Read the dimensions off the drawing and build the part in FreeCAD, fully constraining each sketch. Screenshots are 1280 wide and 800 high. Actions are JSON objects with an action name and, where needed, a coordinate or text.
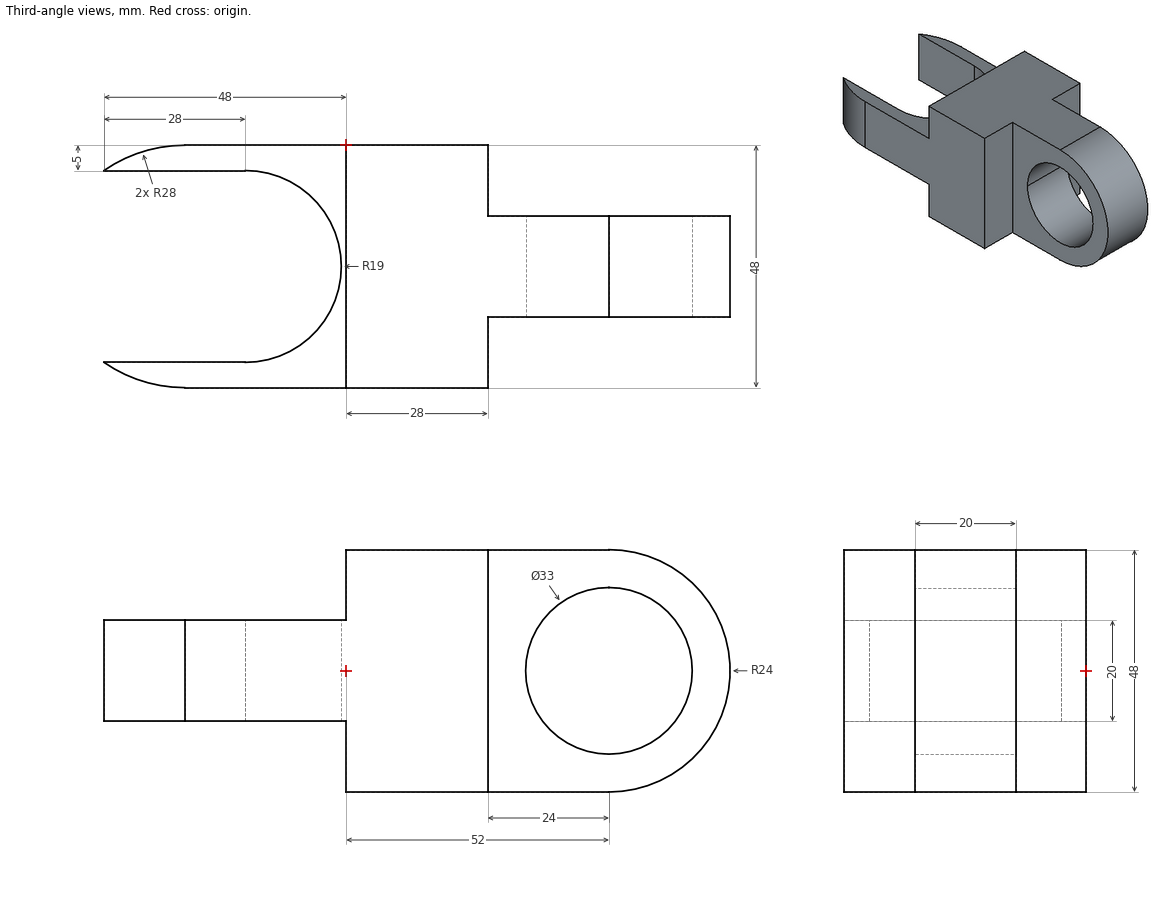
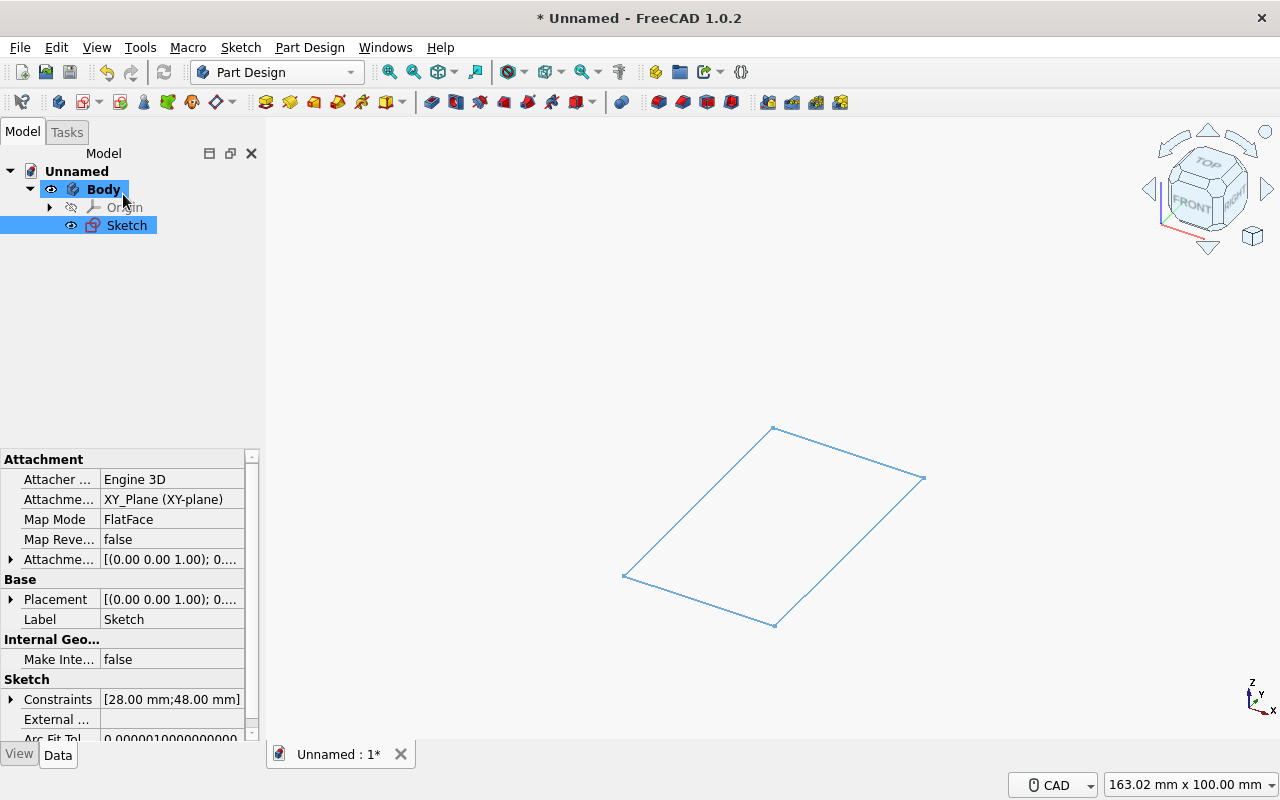
{"action": "left_click", "coordinate": [266, 102]}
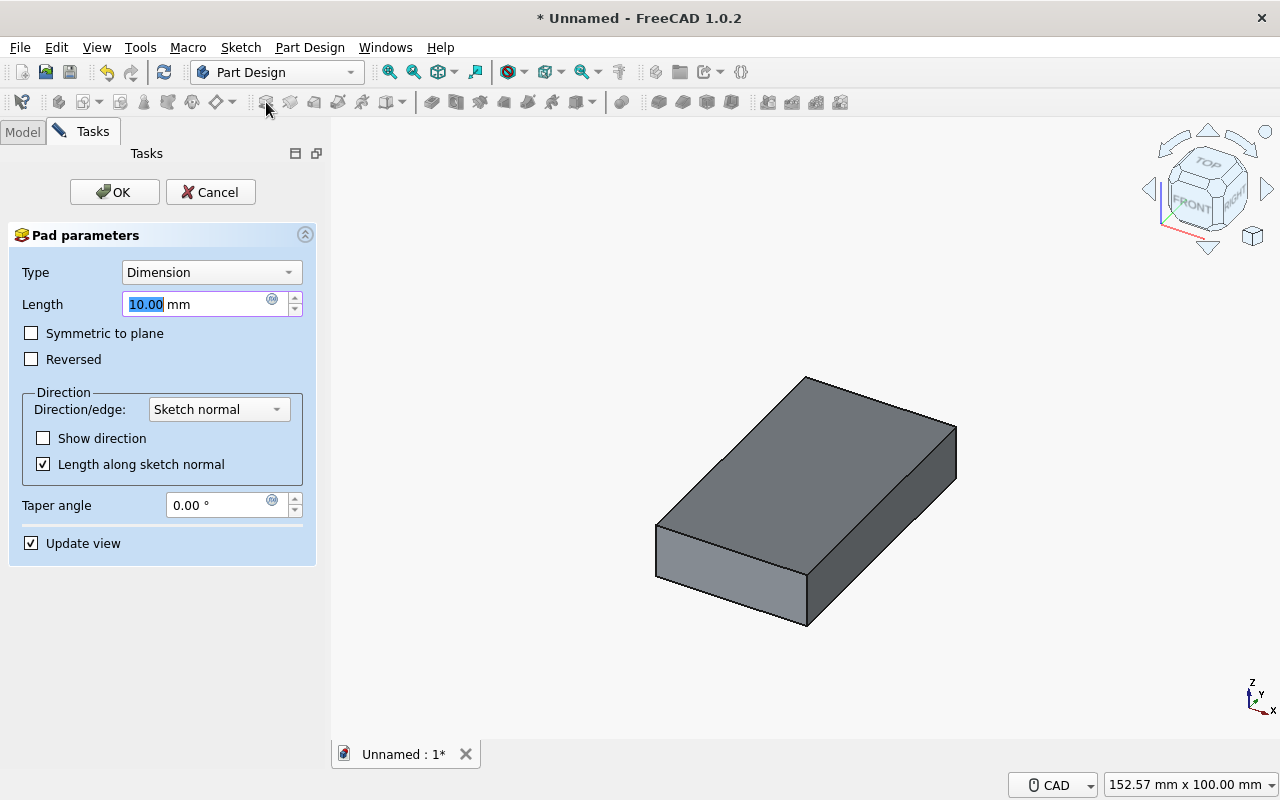
{"action": "type", "text": "48"}
{"action": "key", "text": "Tab"}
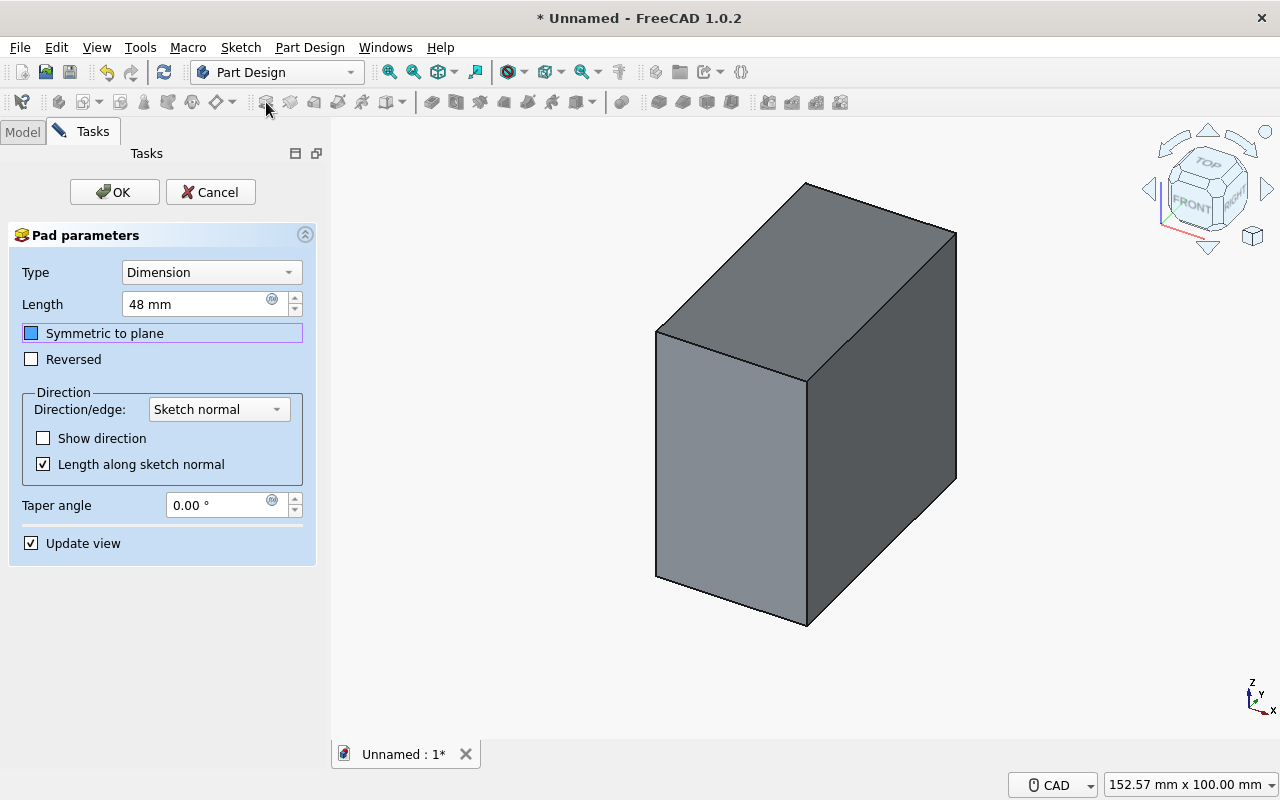
{"action": "left_click", "coordinate": [30, 333]}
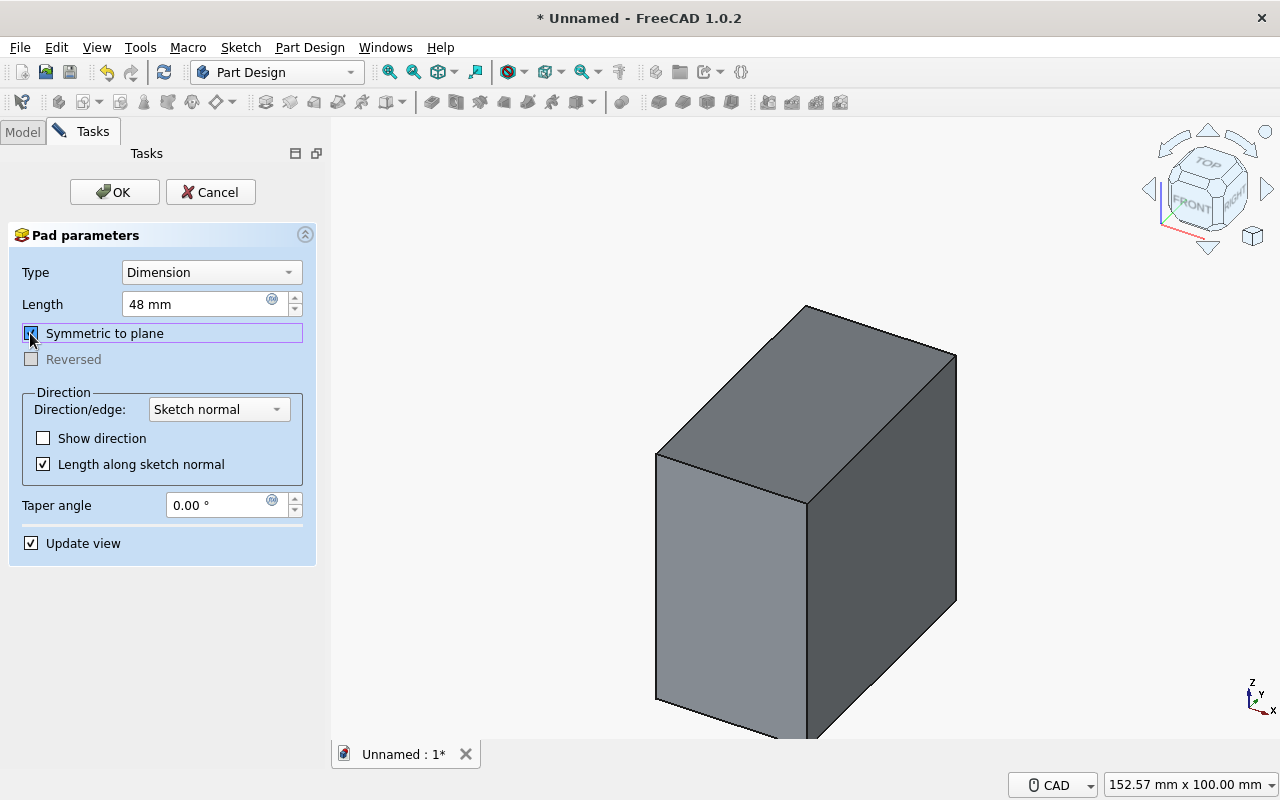
{"action": "left_click", "coordinate": [115, 192]}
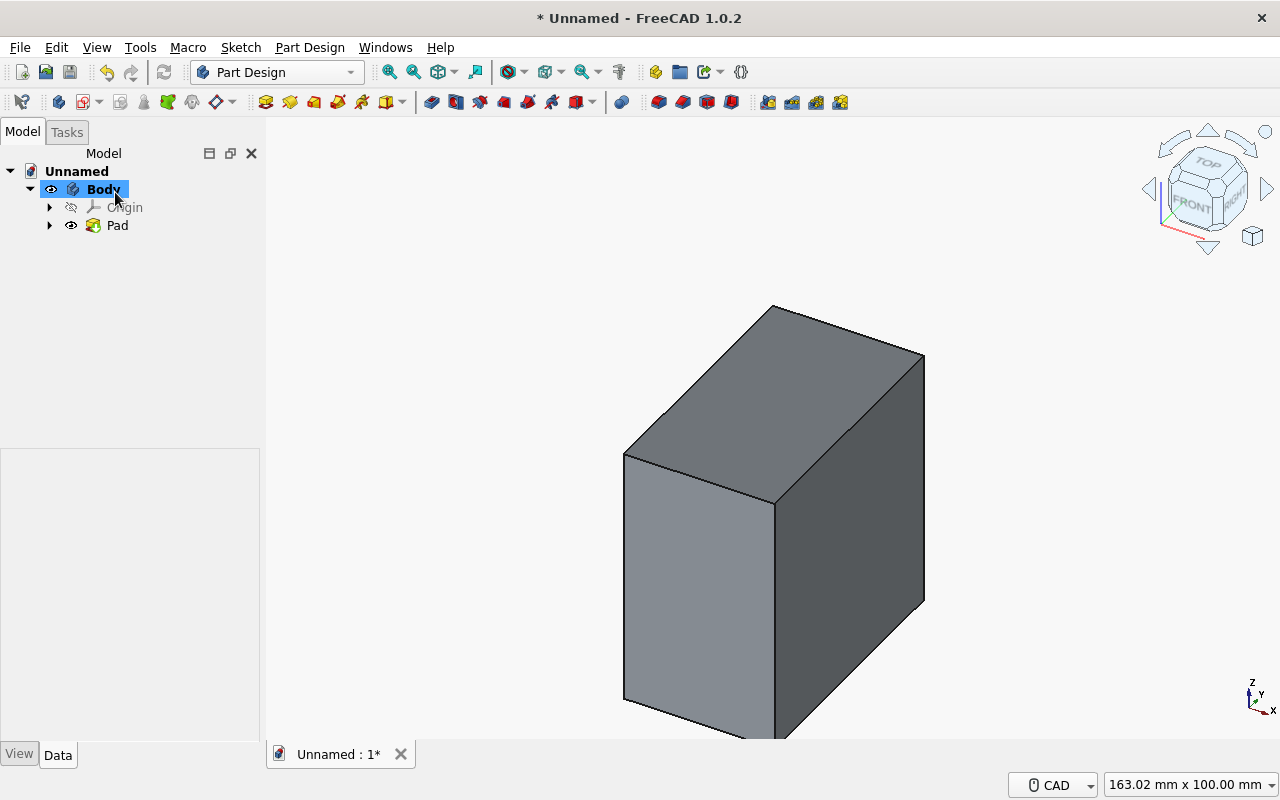
{"action": "left_click", "coordinate": [390, 72]}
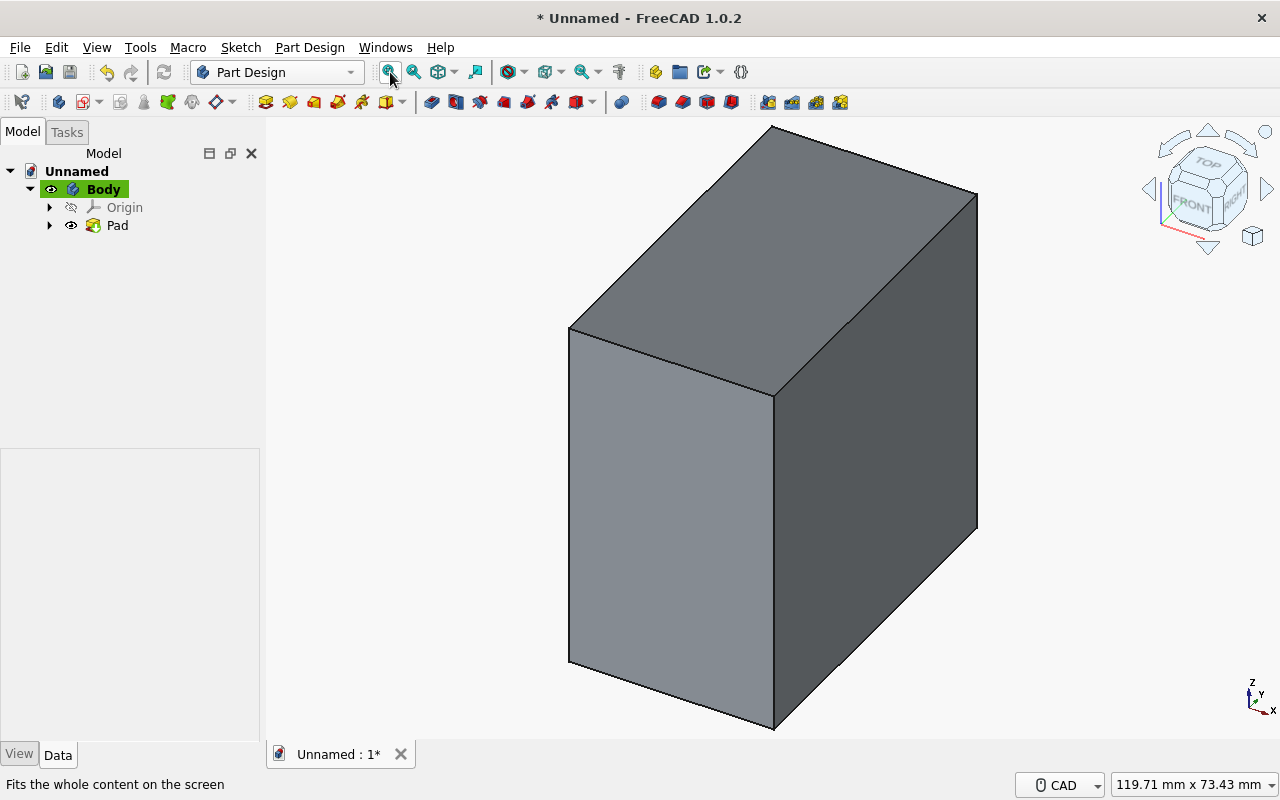
{"action": "left_click", "coordinate": [50, 207]}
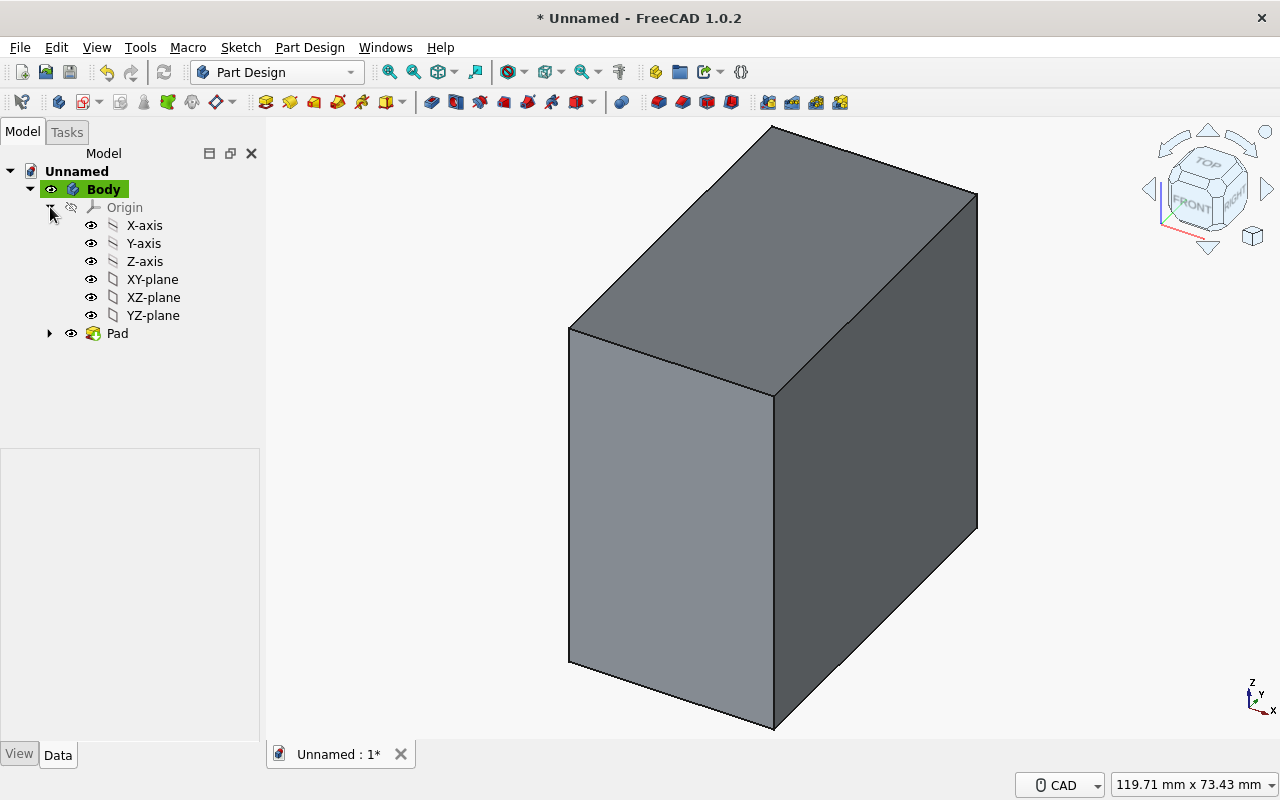
{"action": "left_click", "coordinate": [136, 297]}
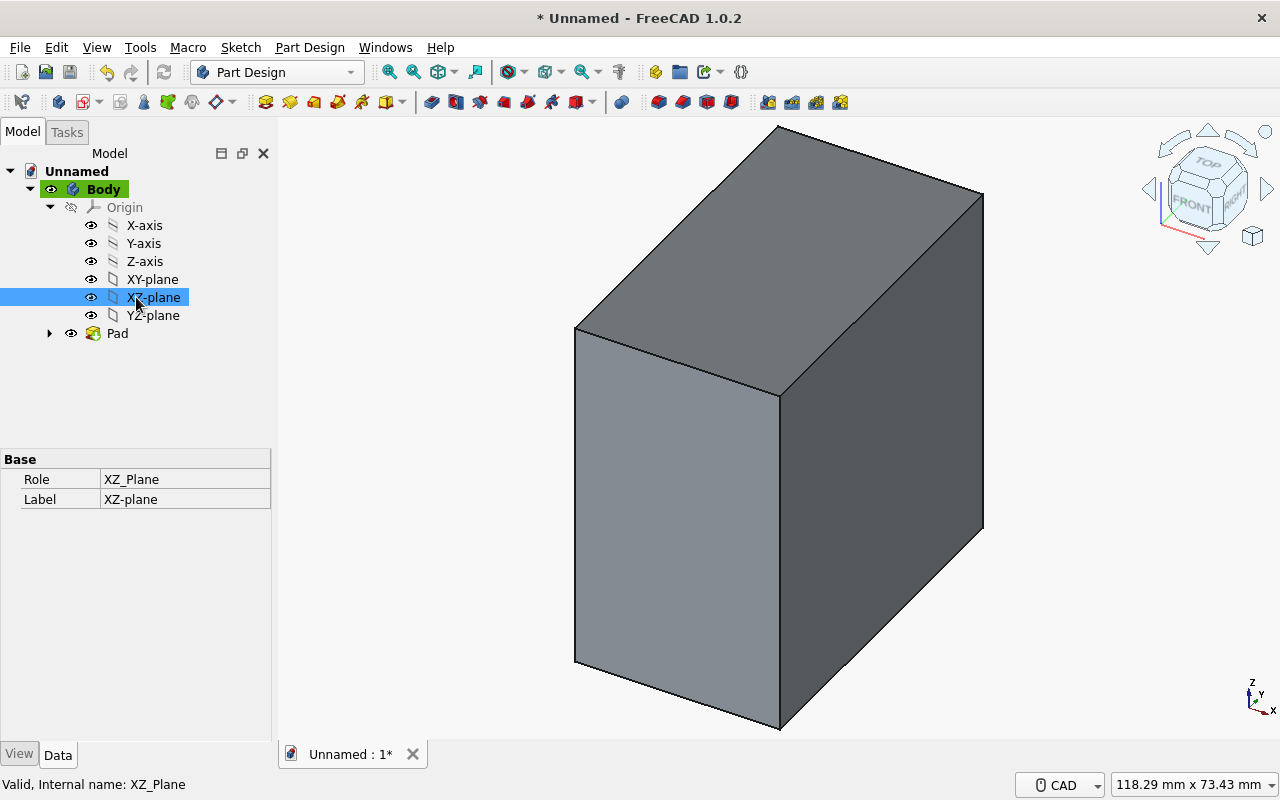
{"action": "left_click", "coordinate": [216, 102]}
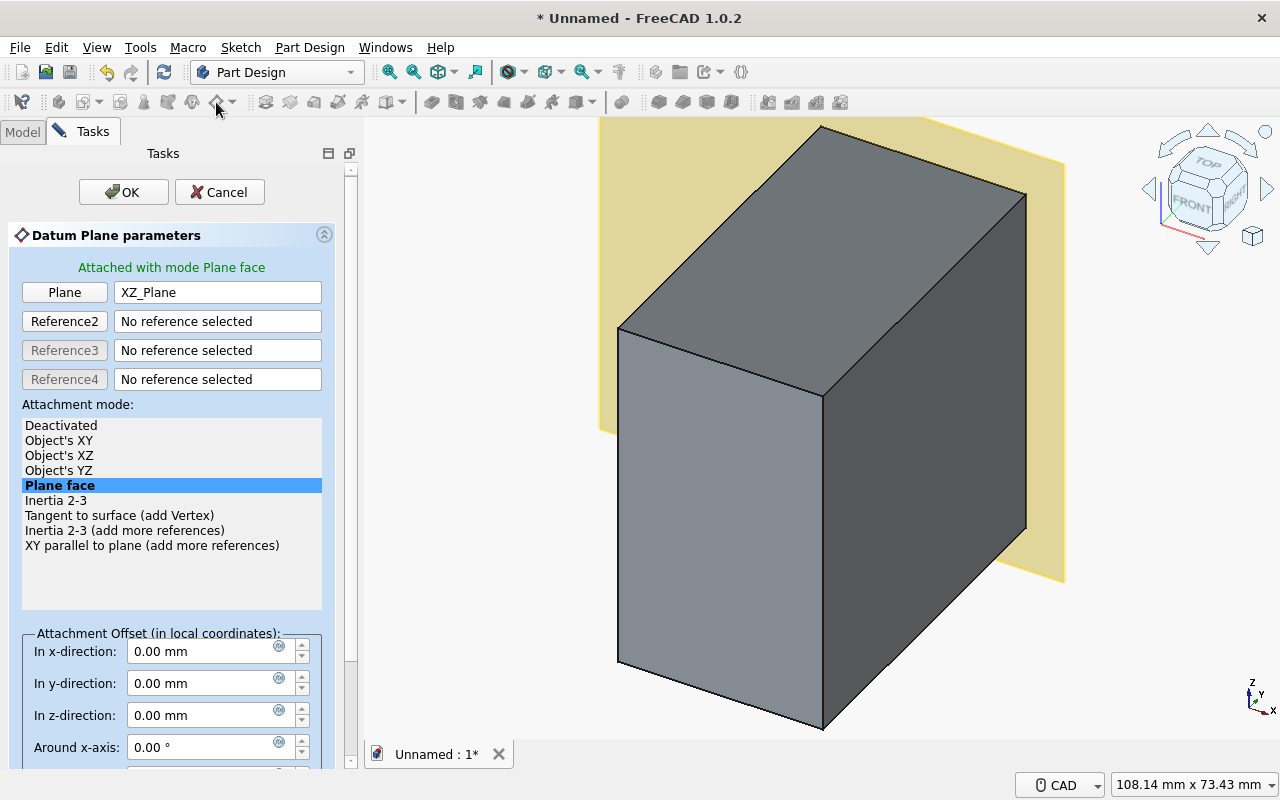
{"action": "triple_click", "coordinate": [210, 715]}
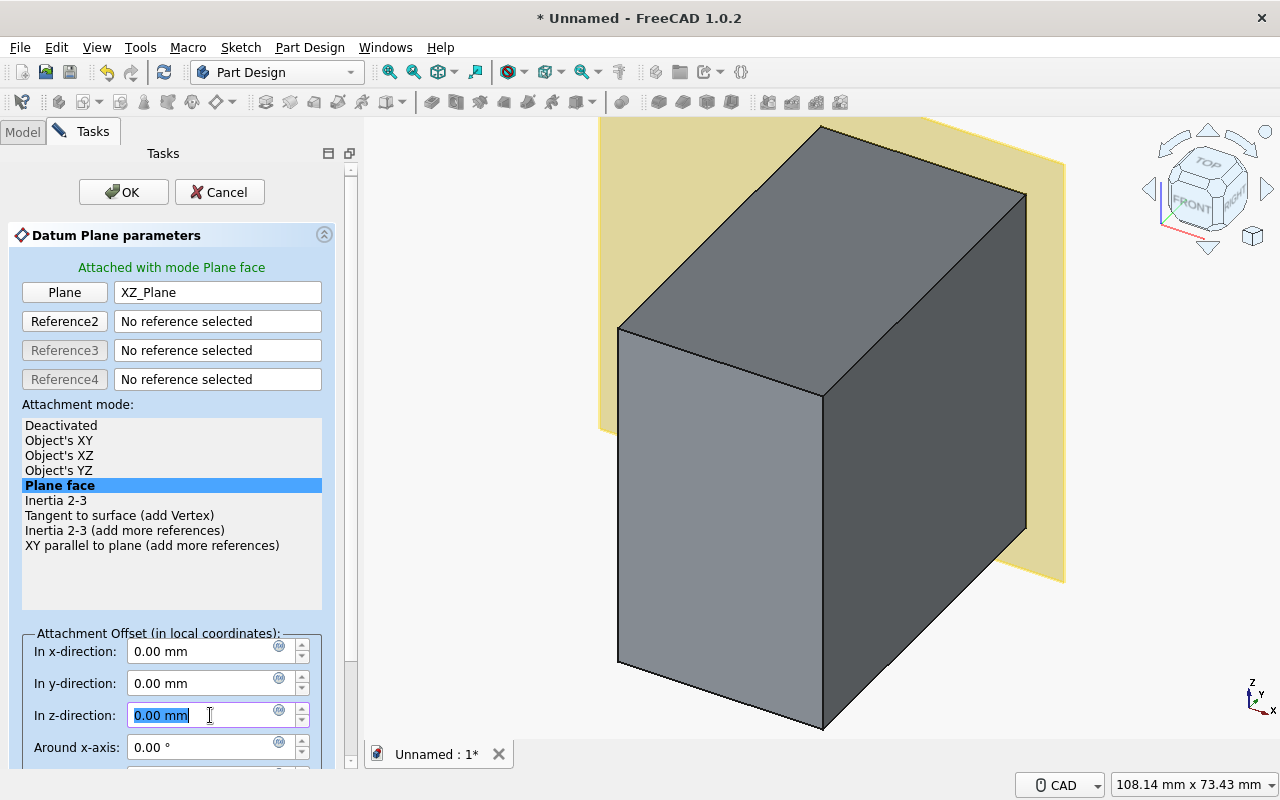
{"action": "type", "text": "24"}
{"action": "key", "text": "Tab"}